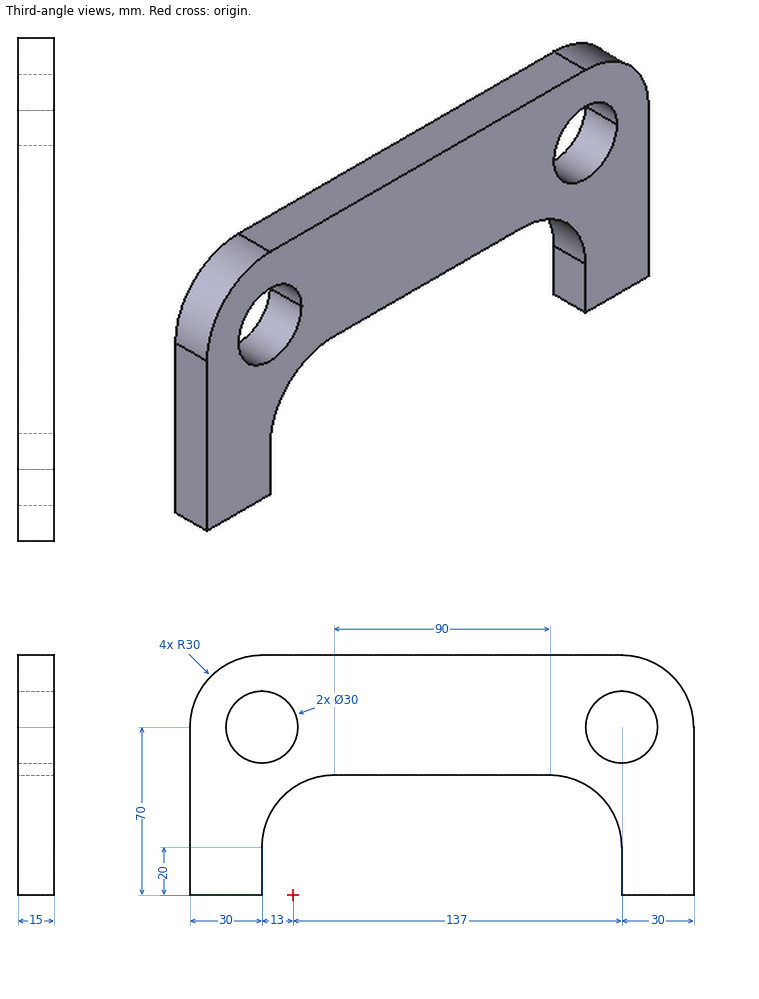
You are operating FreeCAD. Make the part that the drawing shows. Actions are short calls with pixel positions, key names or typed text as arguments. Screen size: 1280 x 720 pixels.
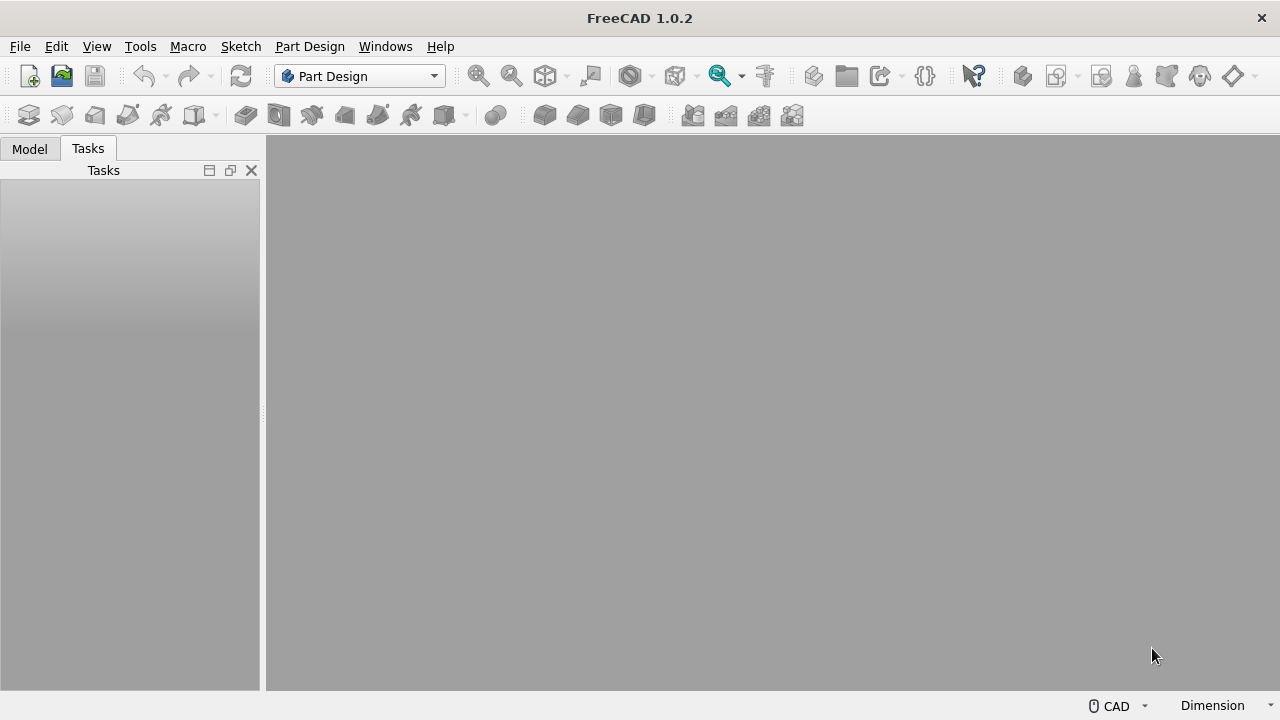
click(29, 76)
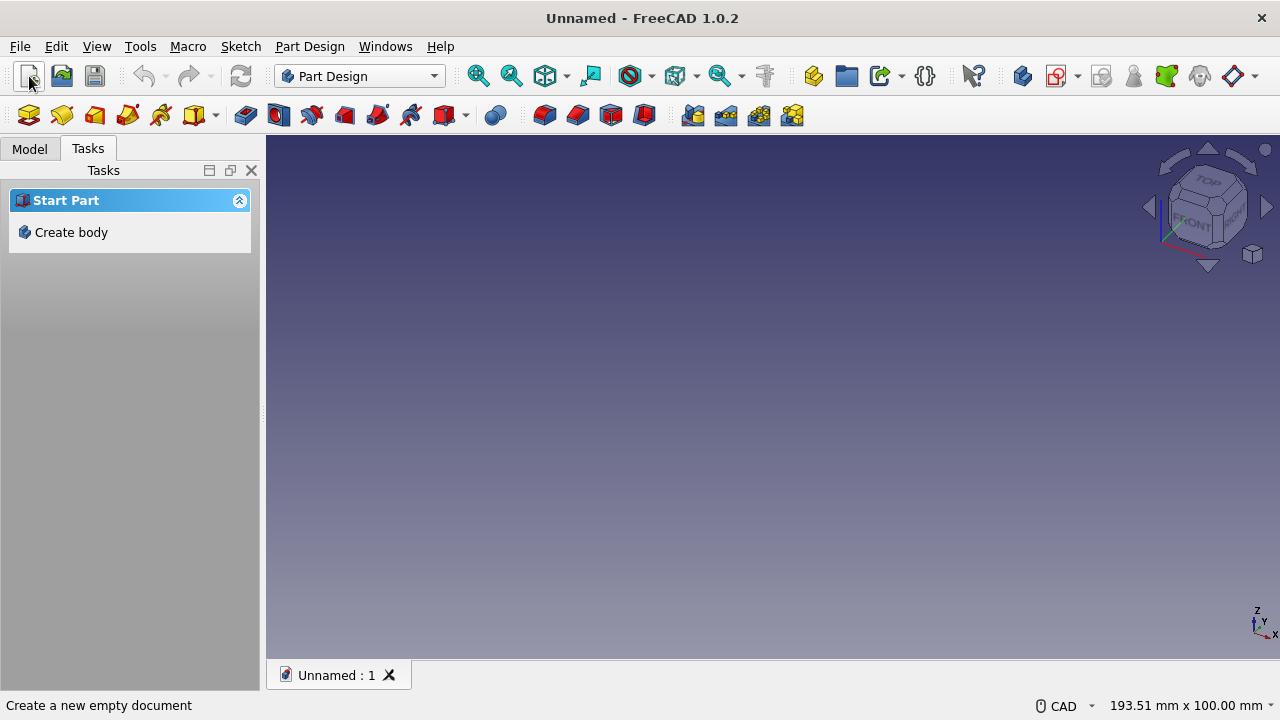
click(1023, 76)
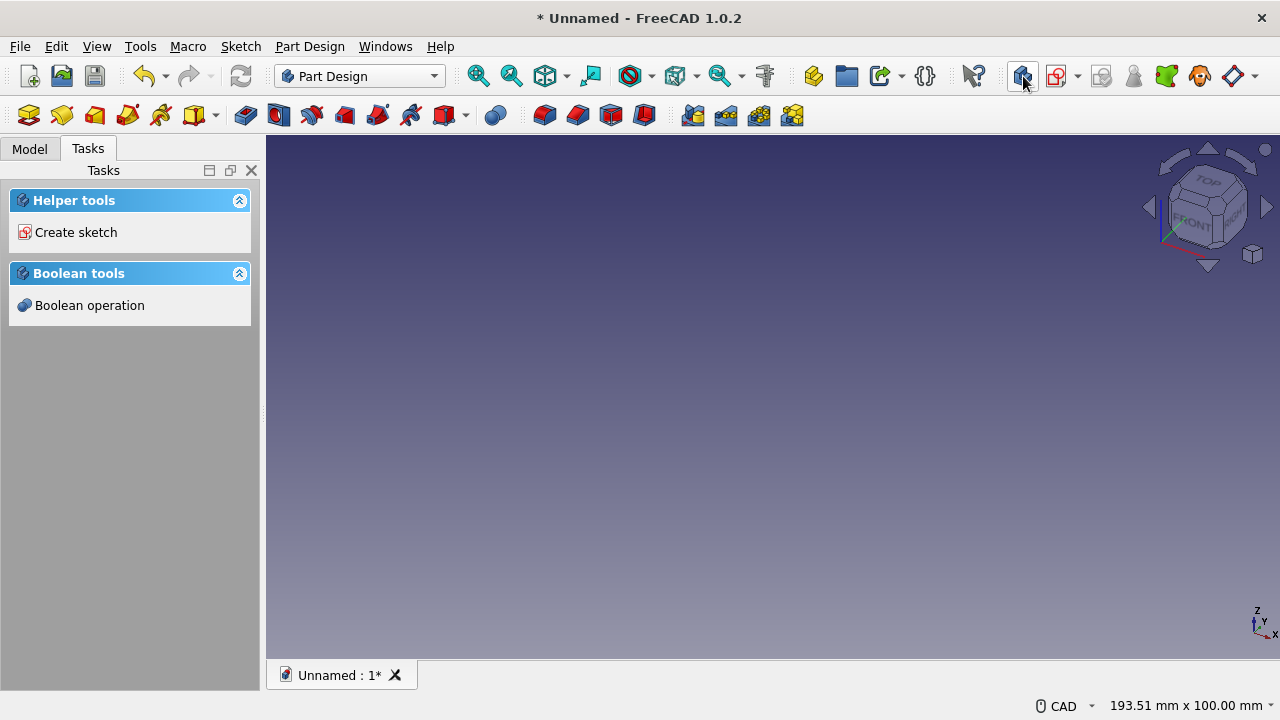
click(30, 148)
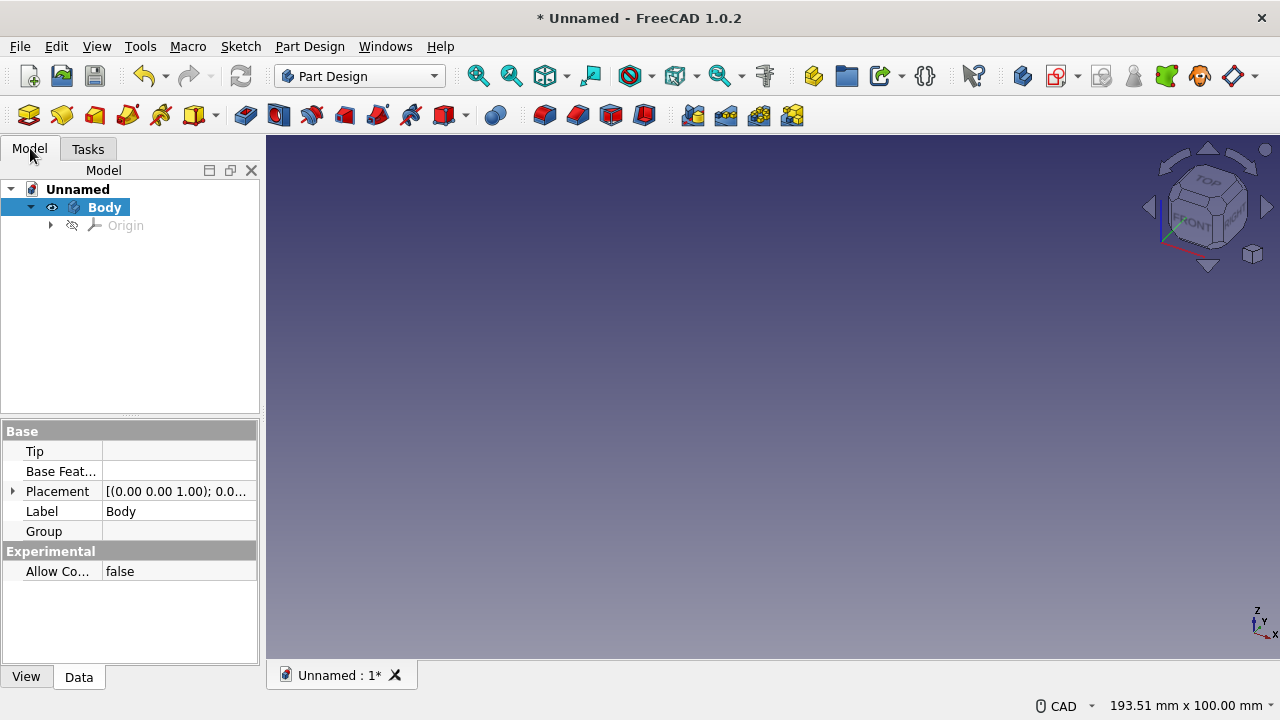
click(51, 225)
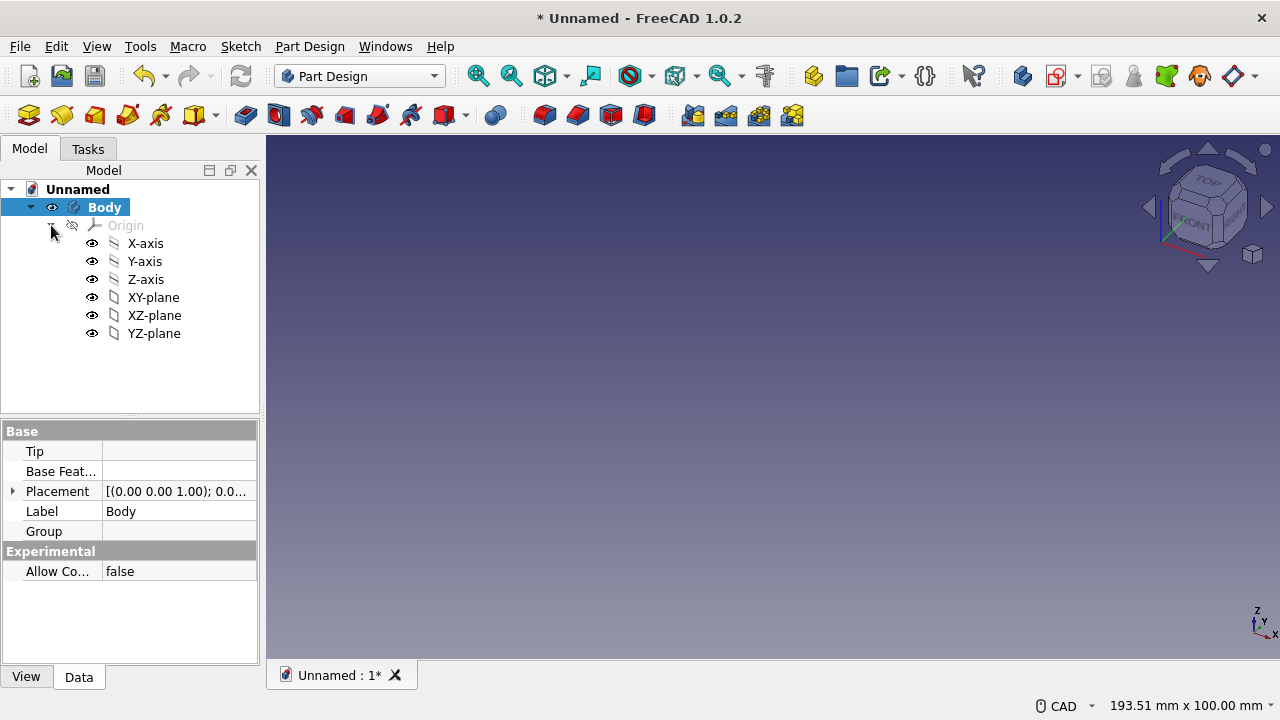
click(137, 333)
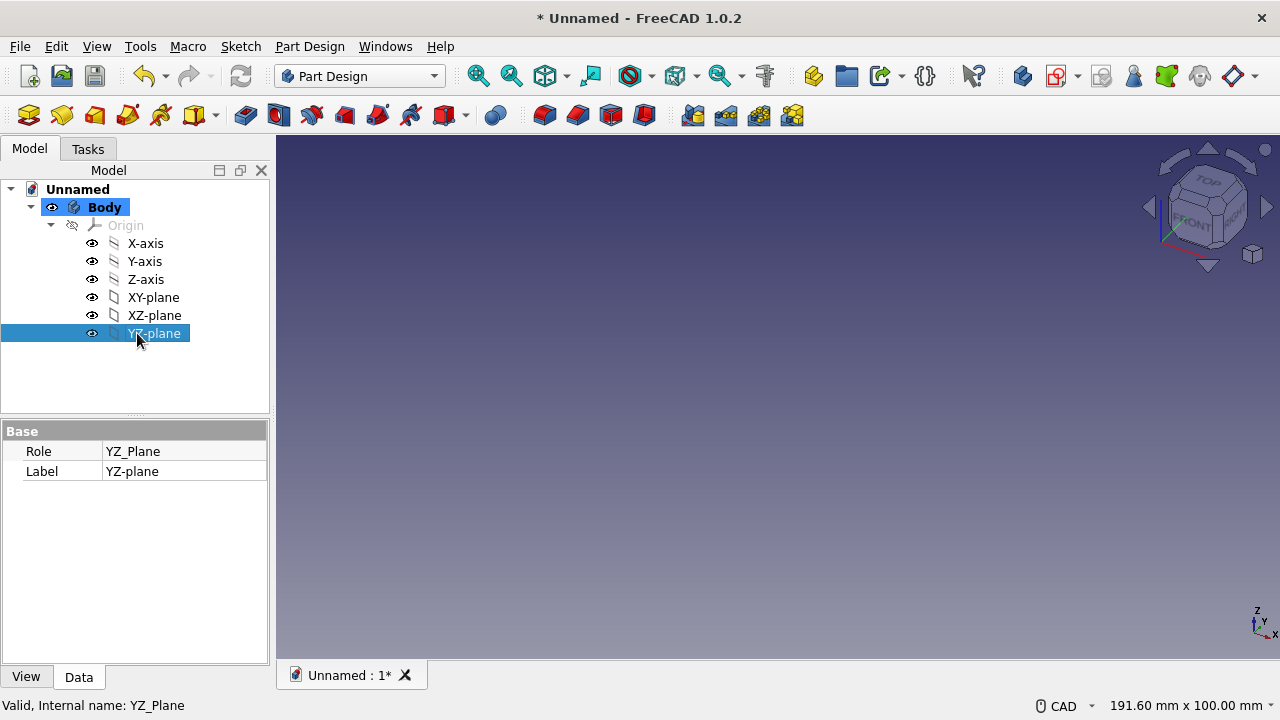
click(1232, 76)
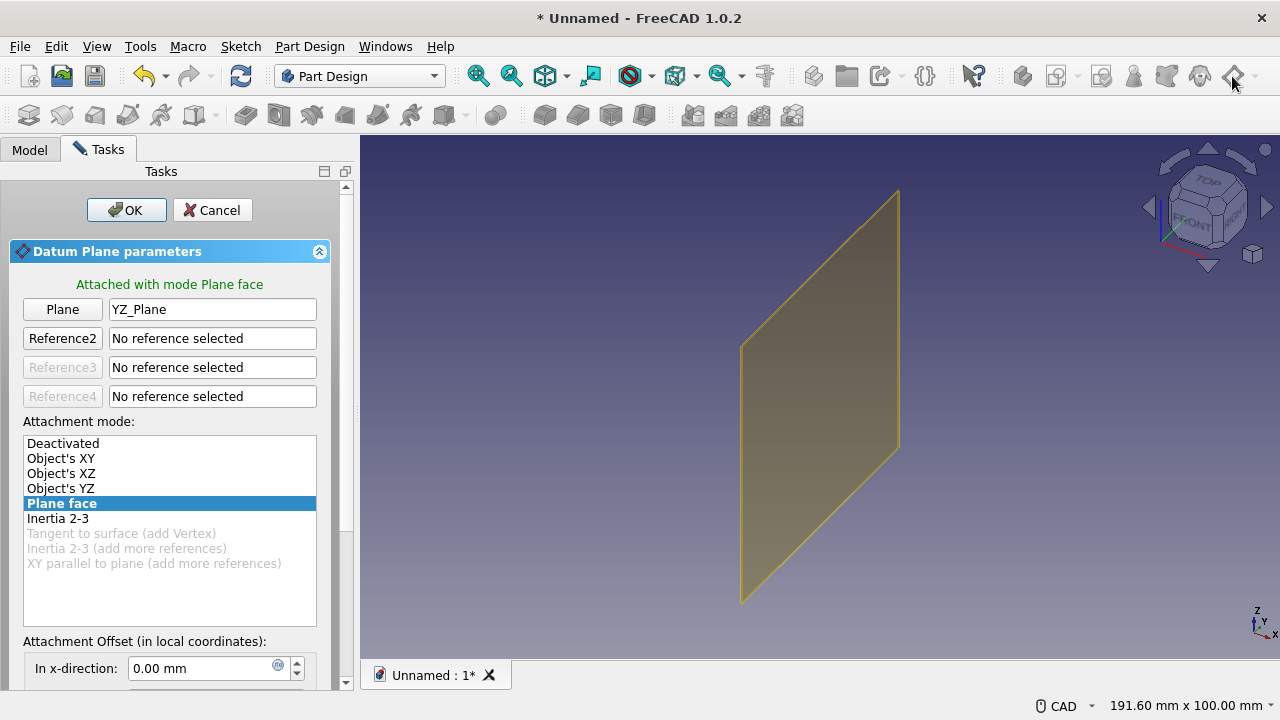
scroll(346, 436, down, 2)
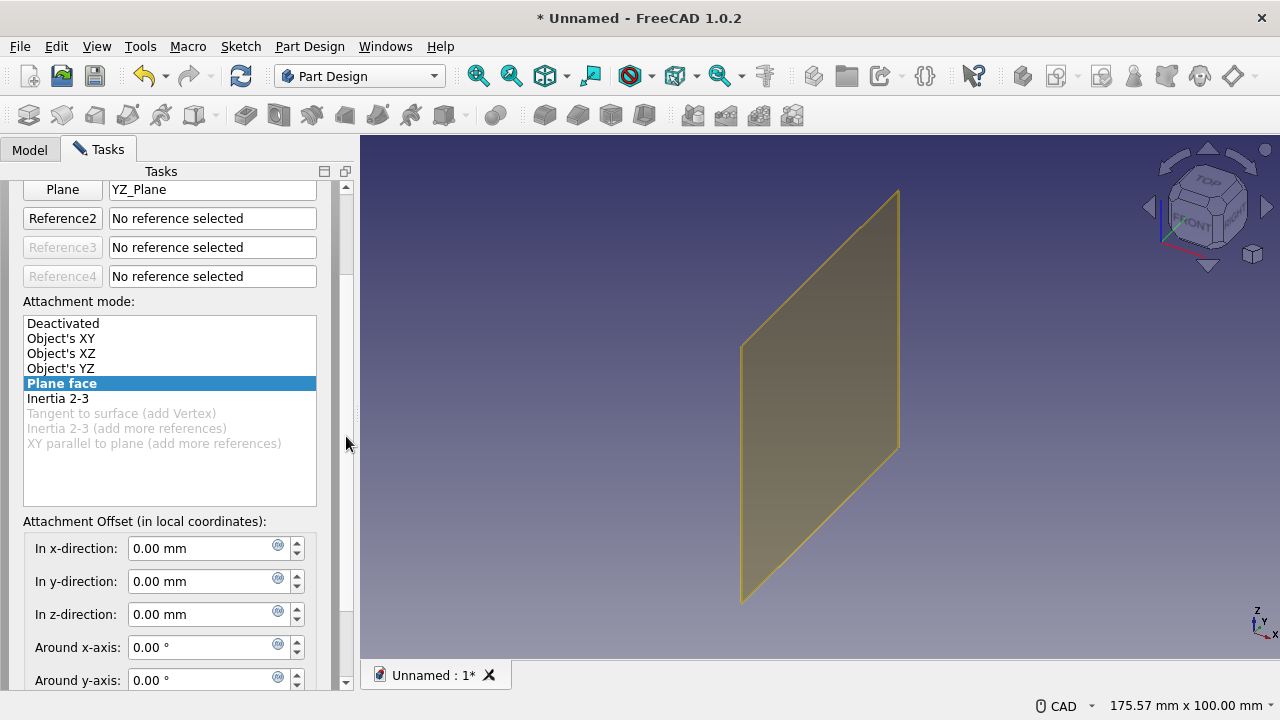
triple_click(210, 614)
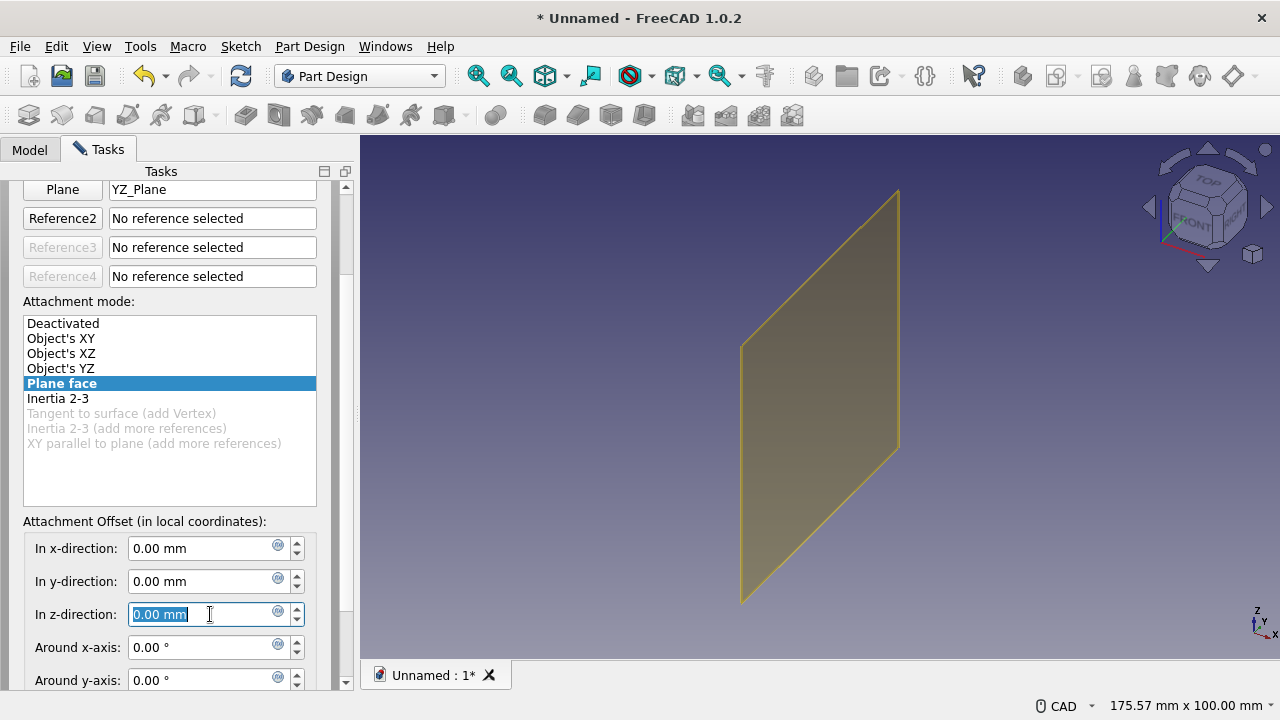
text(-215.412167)
key(Tab)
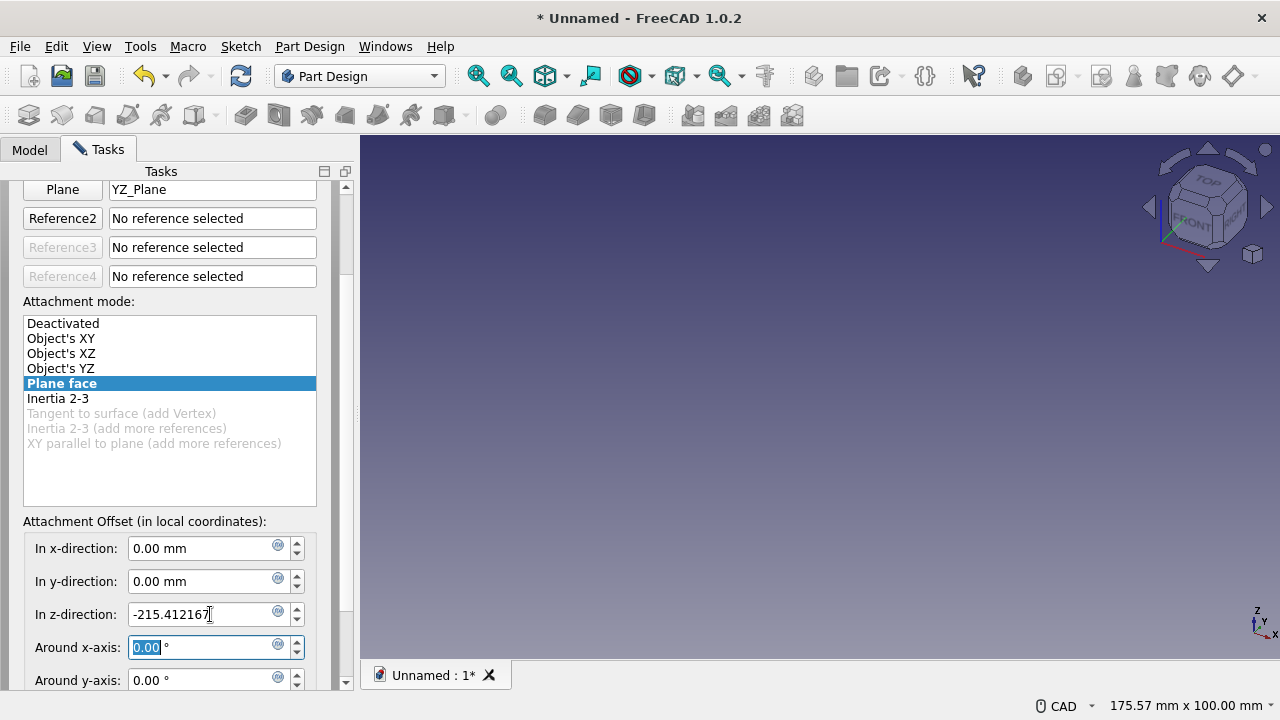
scroll(346, 436, up, 3)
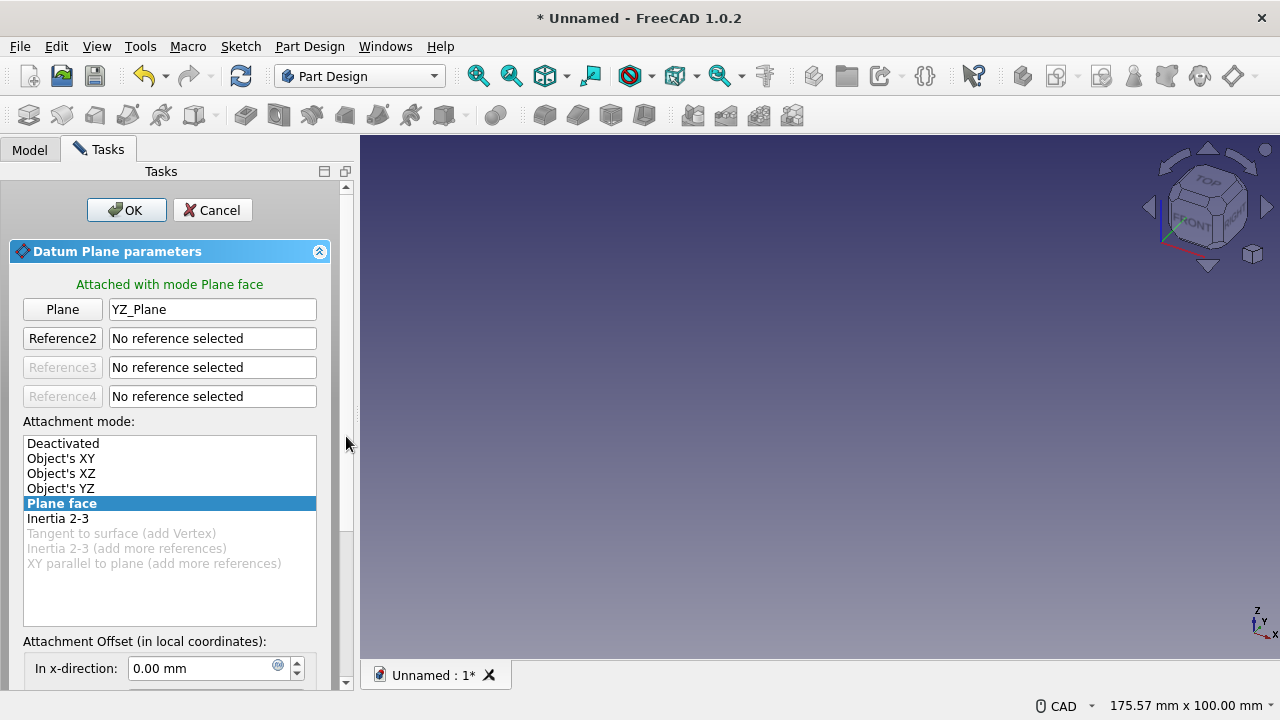
click(127, 210)